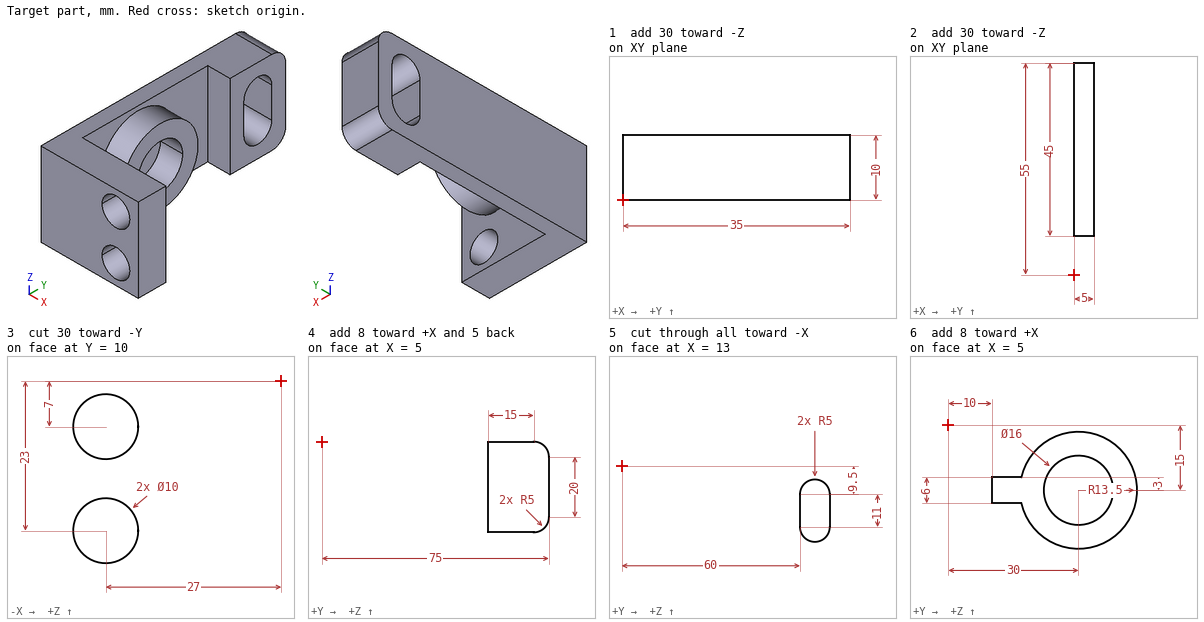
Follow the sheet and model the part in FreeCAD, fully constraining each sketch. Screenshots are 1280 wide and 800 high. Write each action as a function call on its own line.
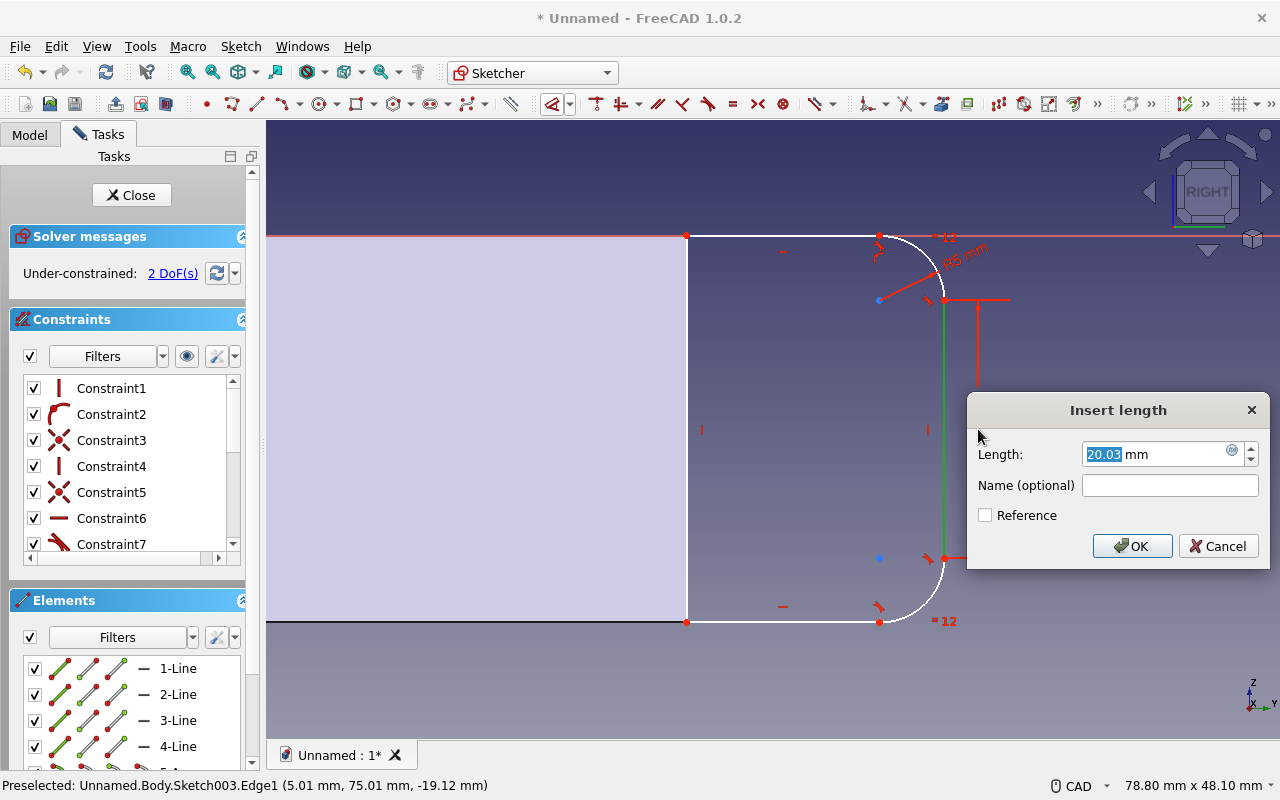
text(20)
key(Return)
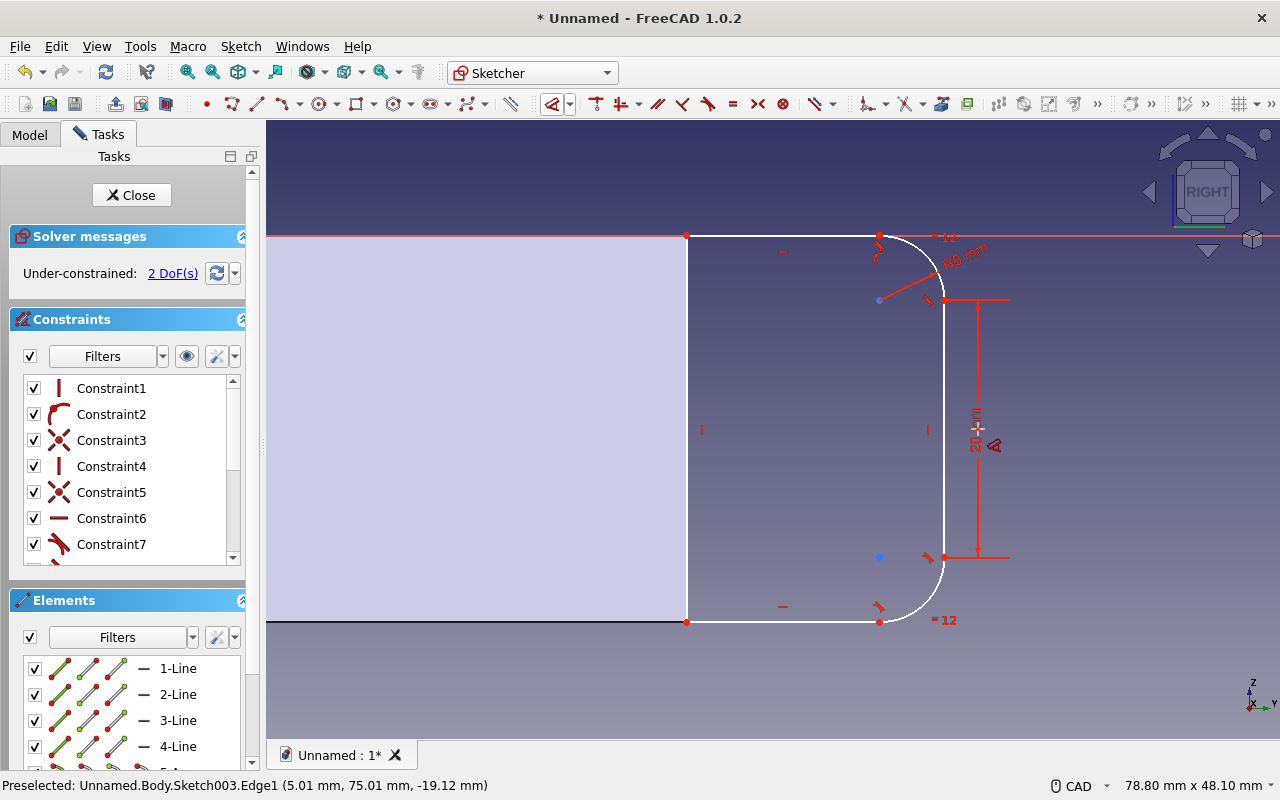
click(822, 236)
click(783, 202)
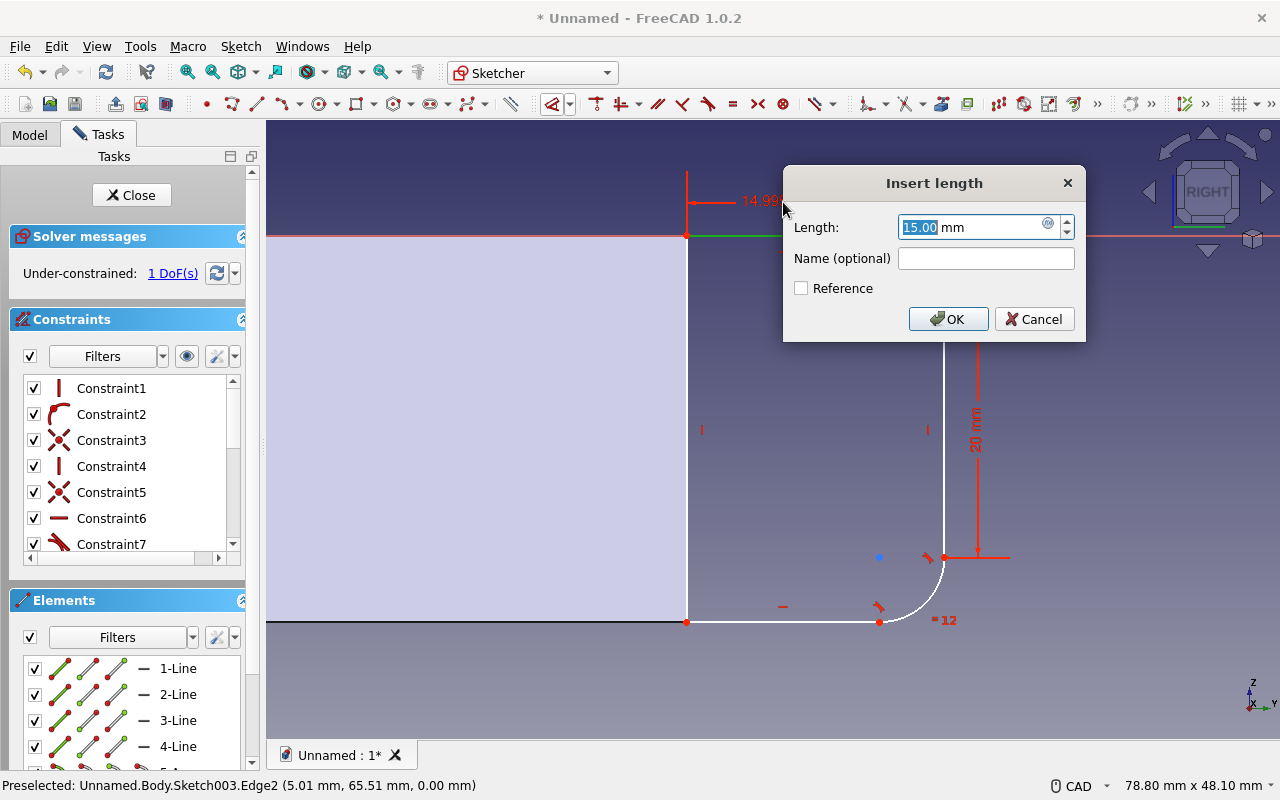
text(15)
key(Return)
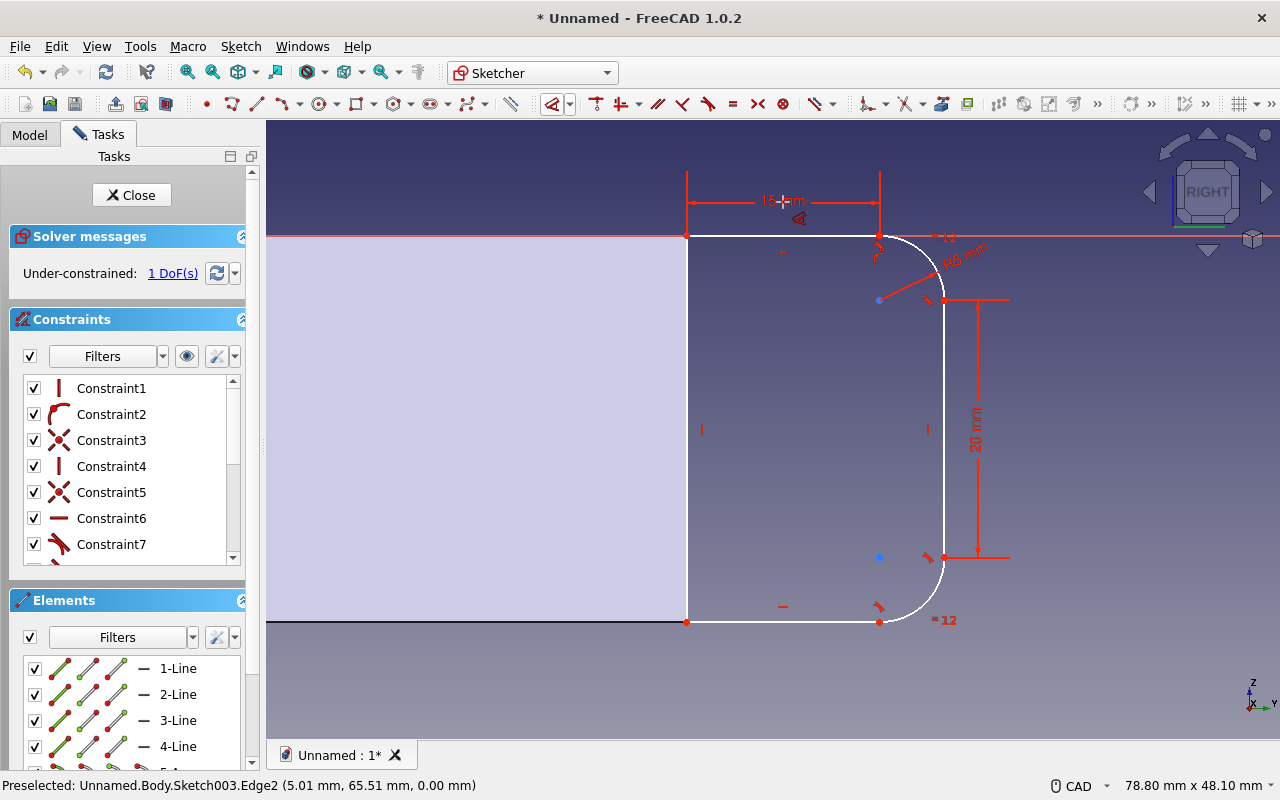
click(944, 558)
click(619, 202)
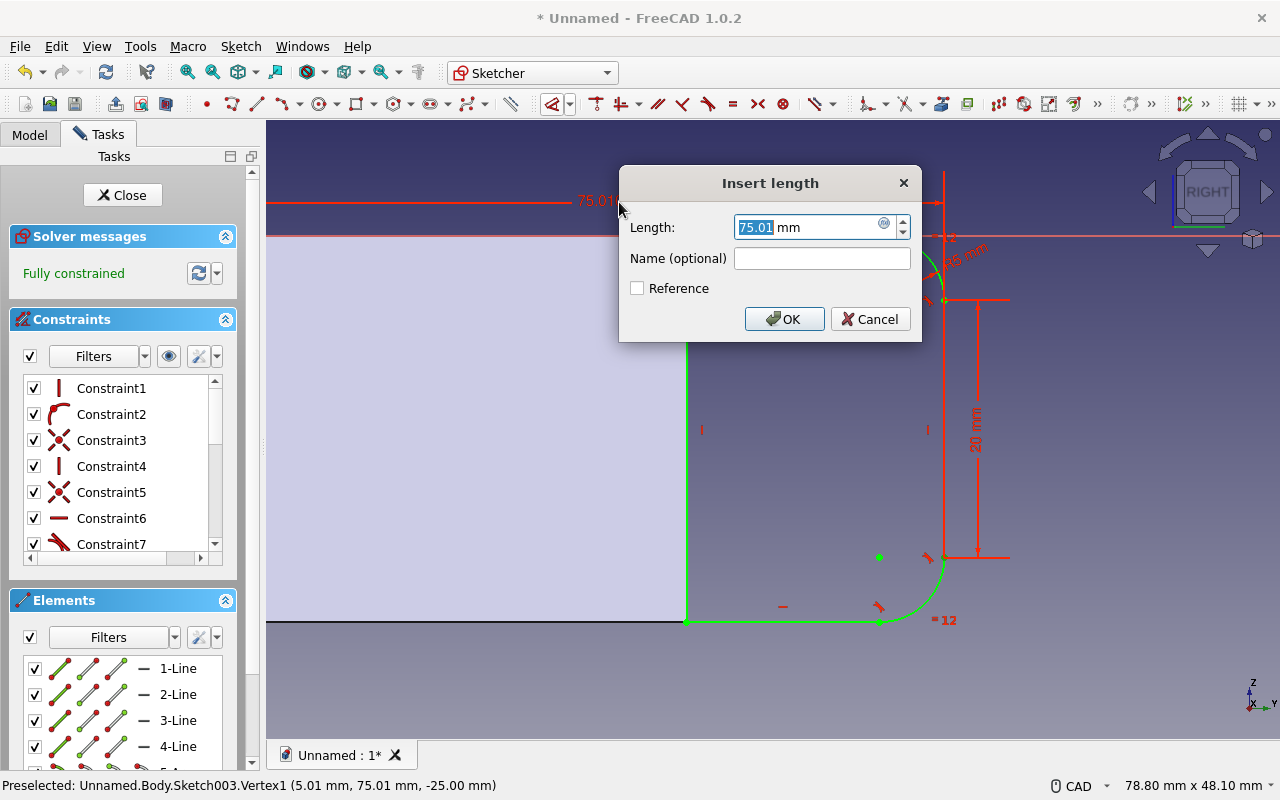
text(75)
key(Return)
key(Escape)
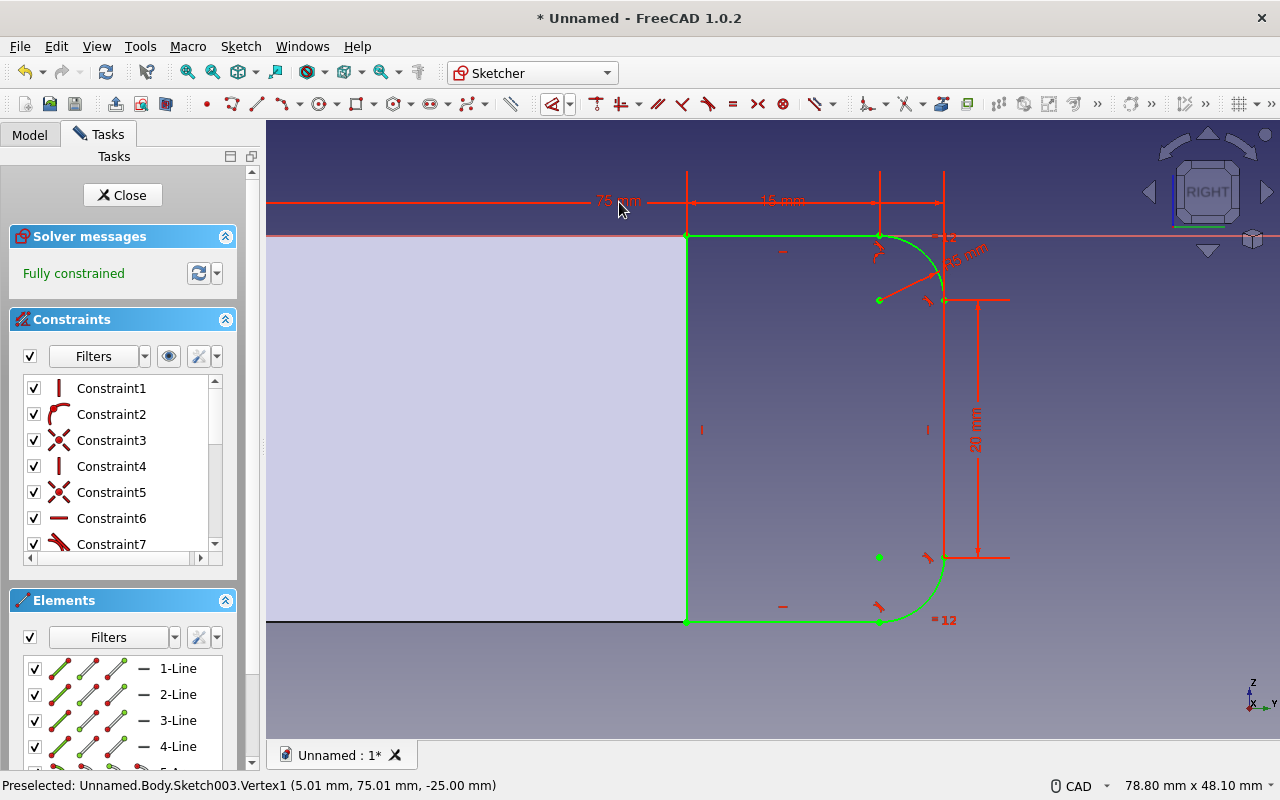
click(123, 195)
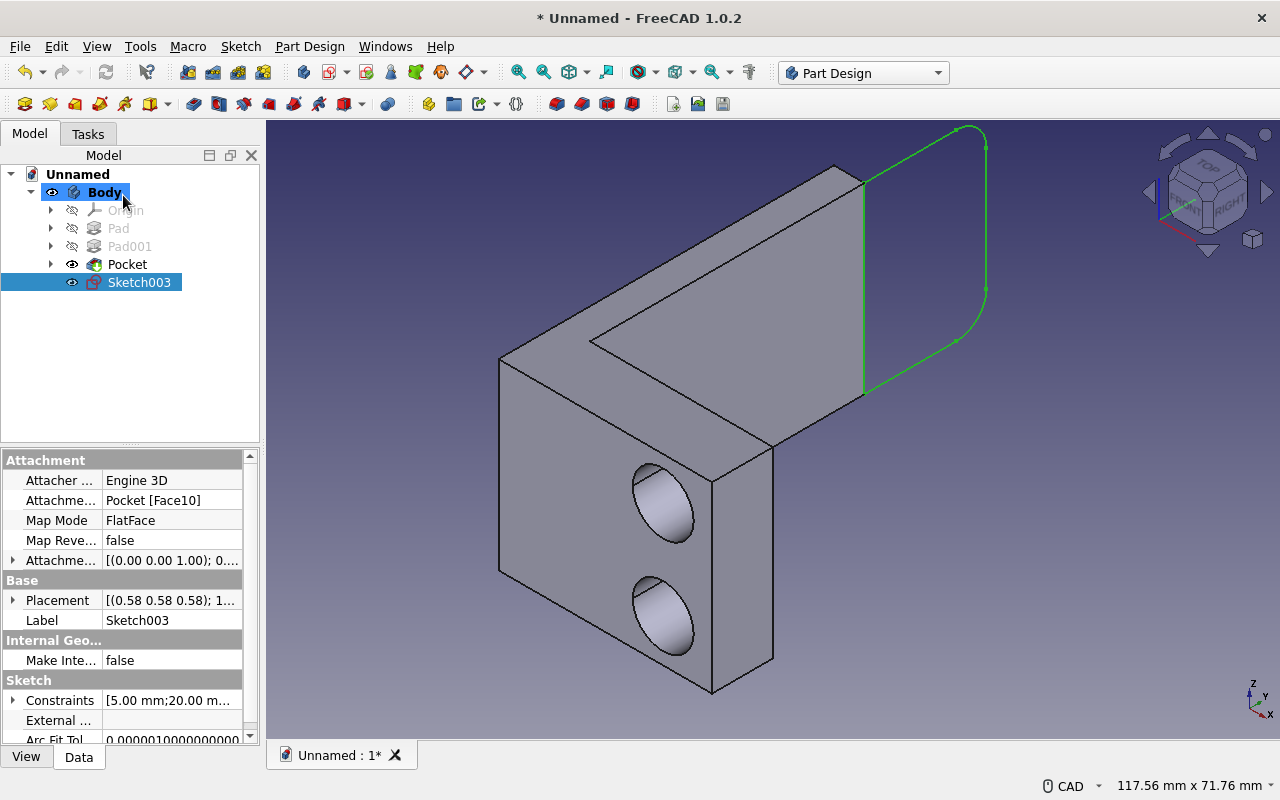
click(25, 104)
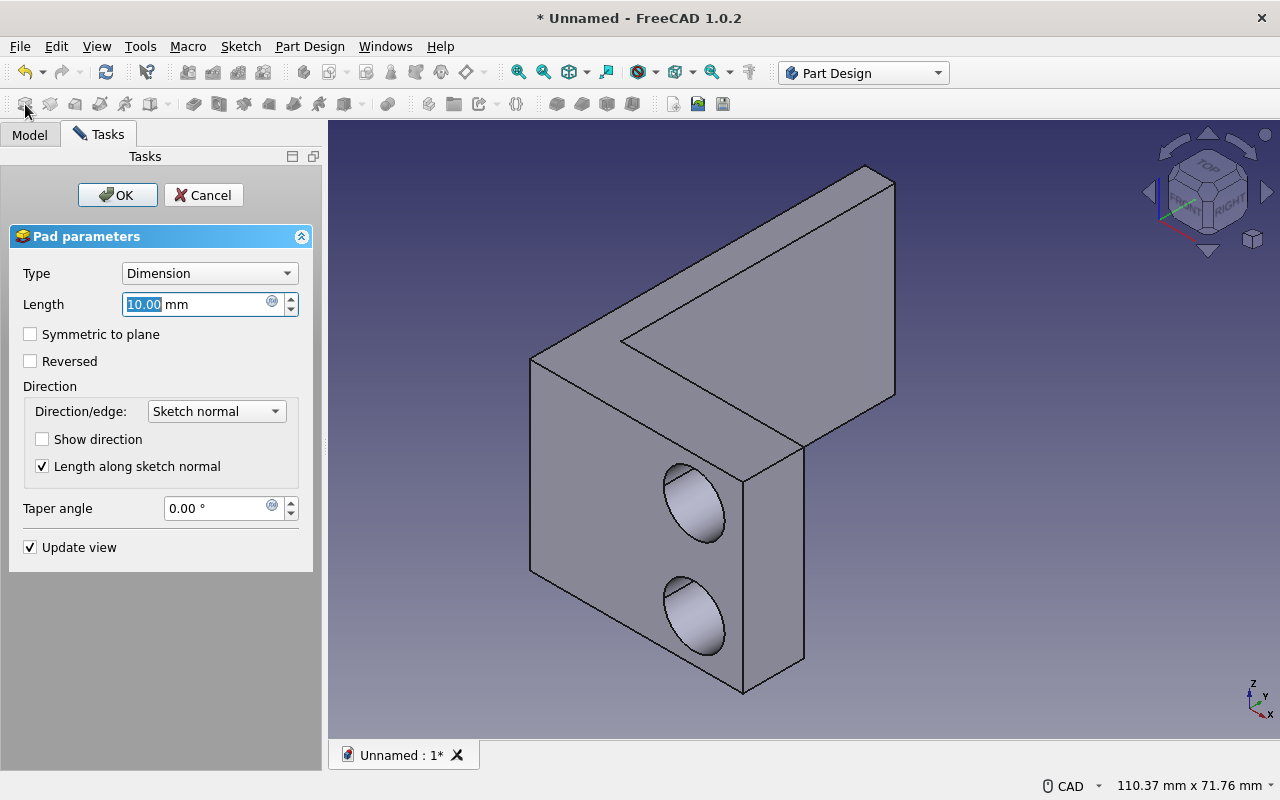
click(210, 274)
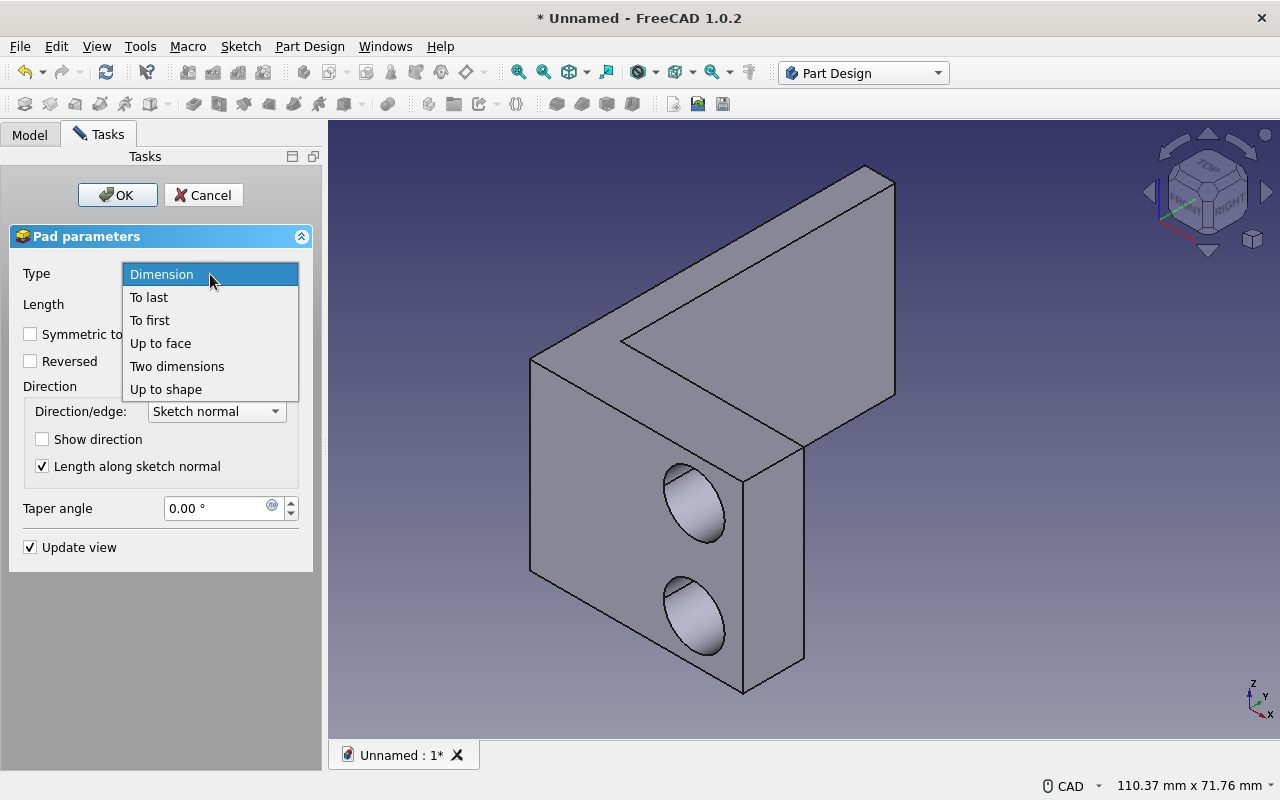
click(208, 366)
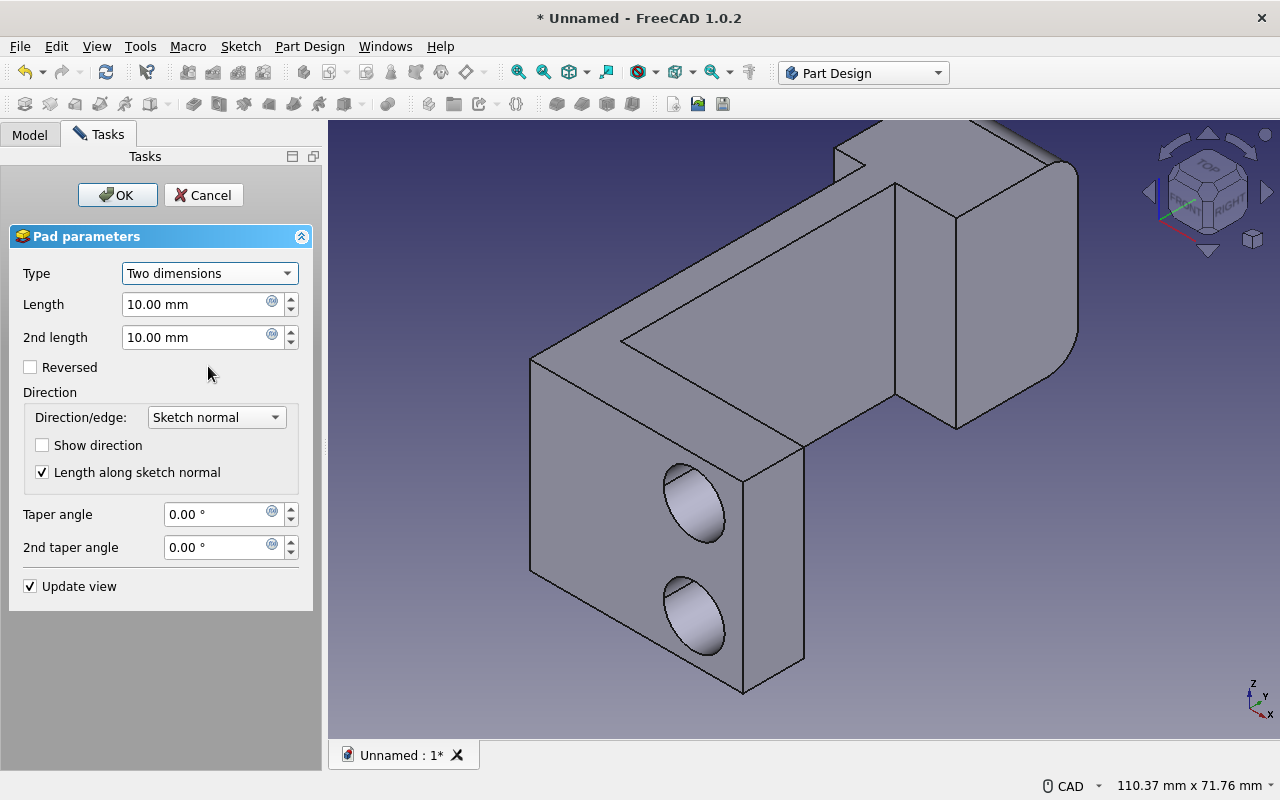
triple_click(204, 304)